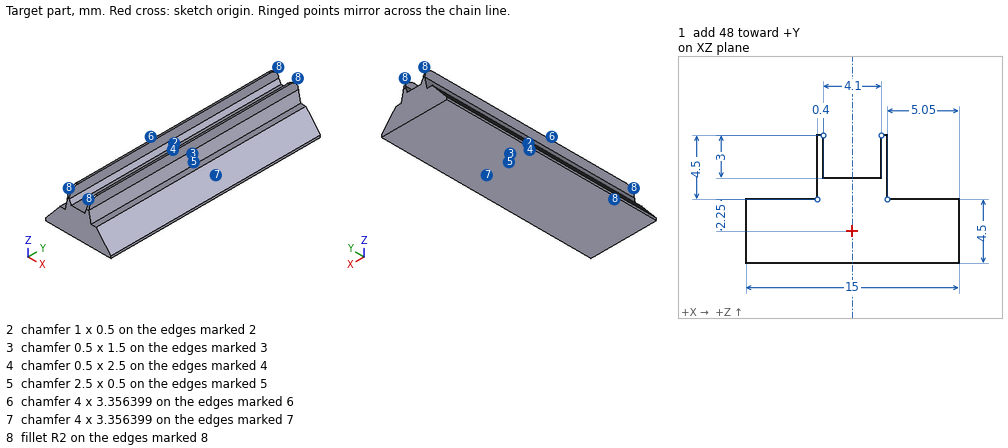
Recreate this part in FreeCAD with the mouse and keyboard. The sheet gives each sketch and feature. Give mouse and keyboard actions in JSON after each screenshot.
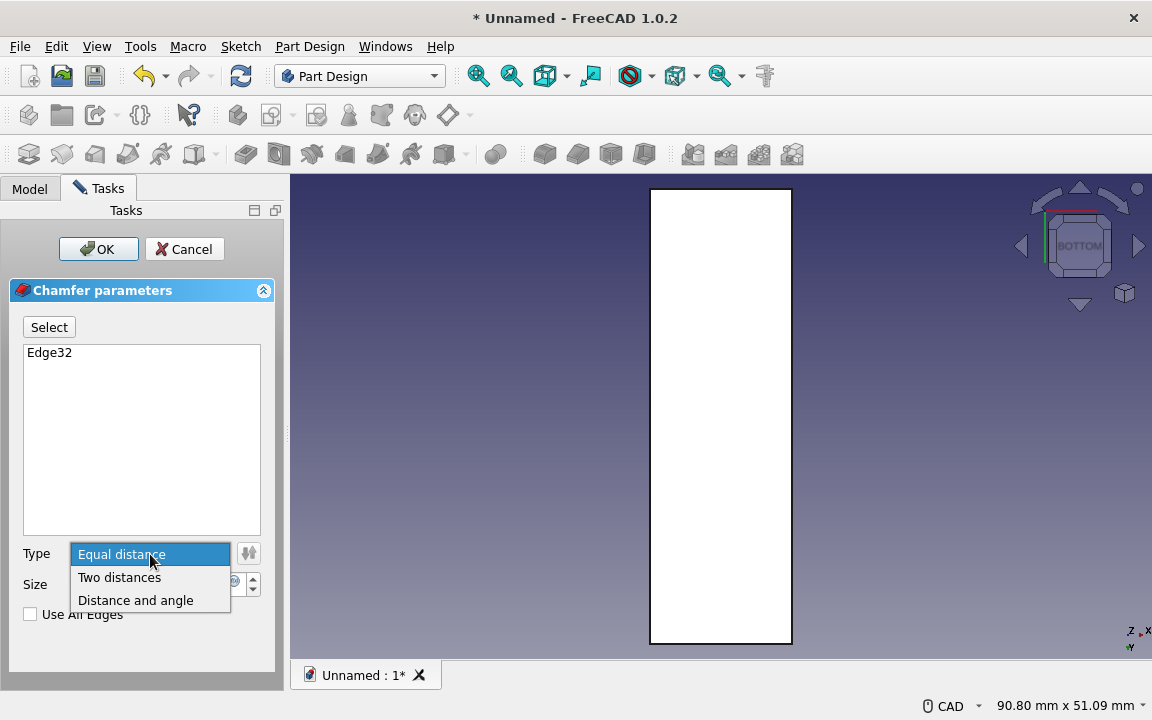
{"action": "left_click", "coordinate": [148, 578]}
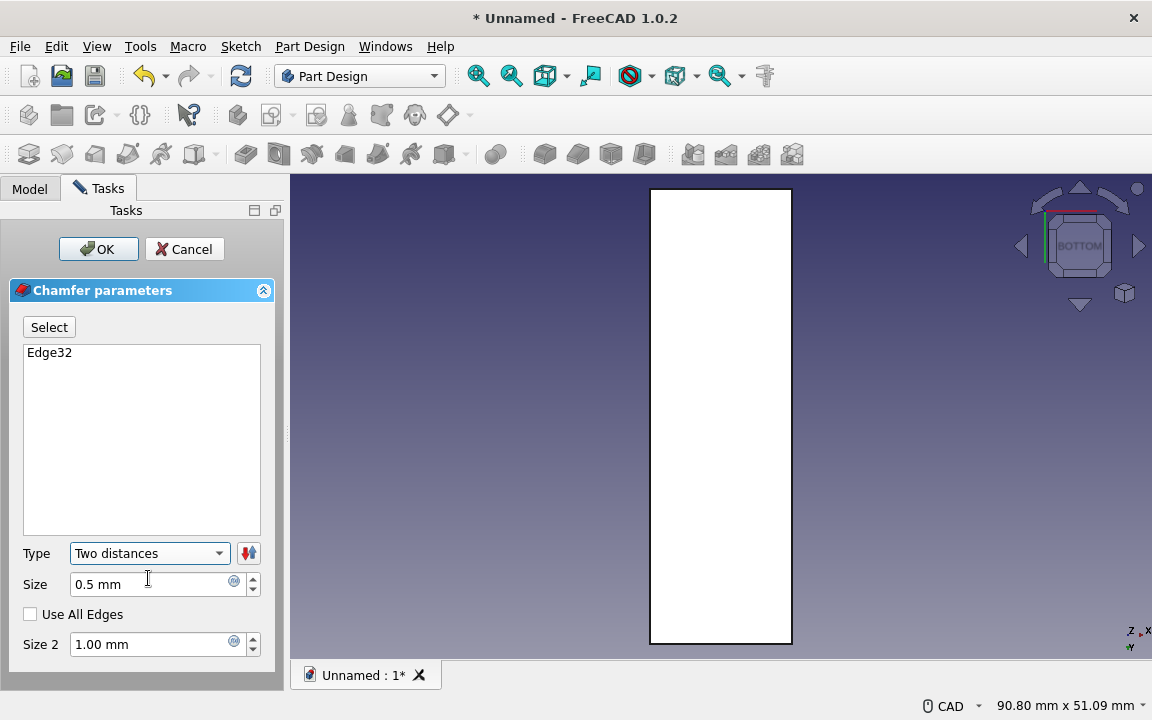
{"action": "triple_click", "coordinate": [158, 644]}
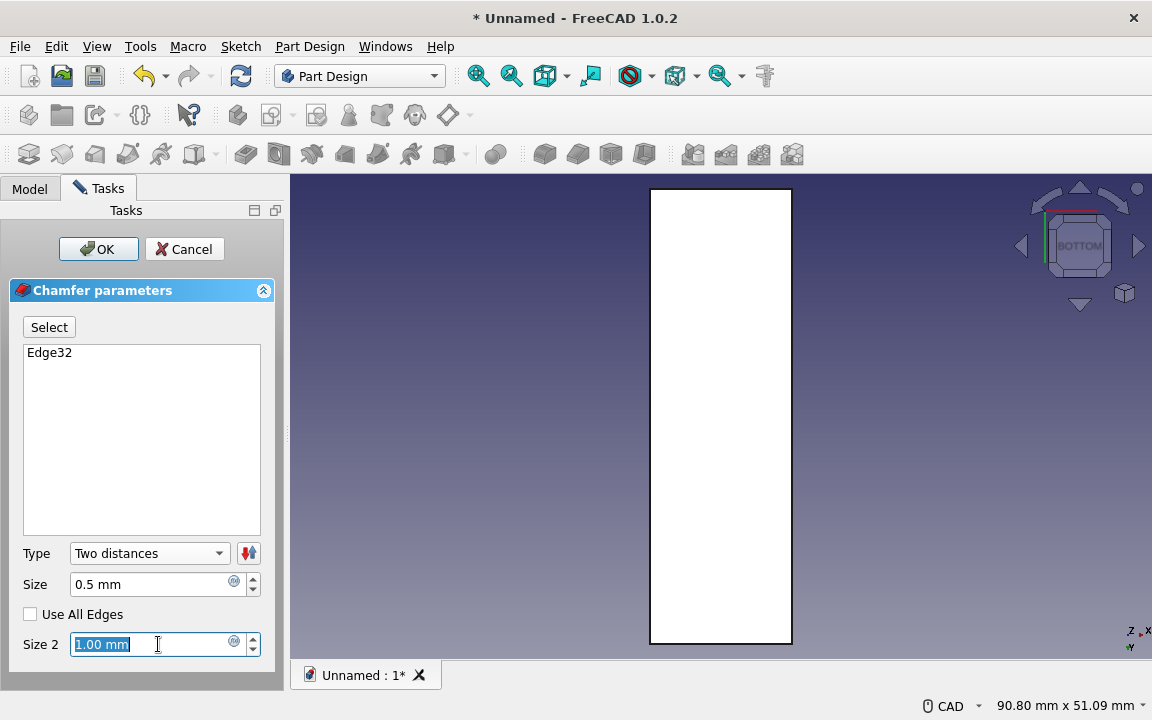
{"action": "type", "text": "2.5"}
{"action": "key", "text": "Tab"}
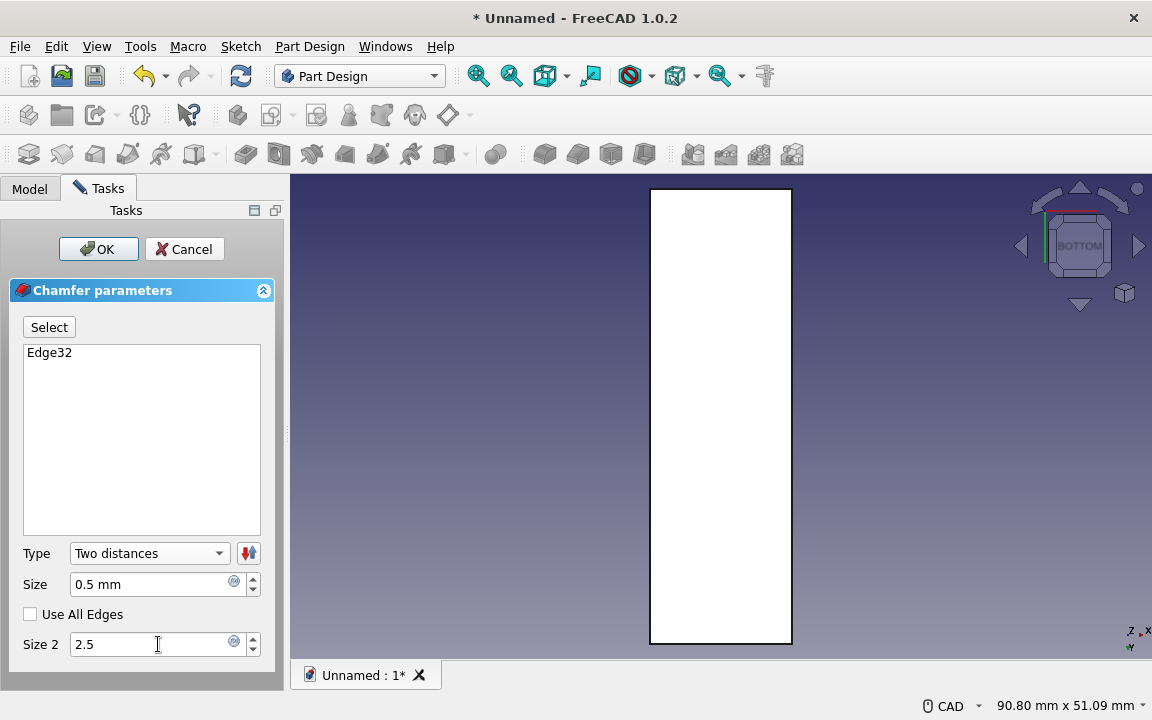
{"action": "left_click", "coordinate": [249, 554]}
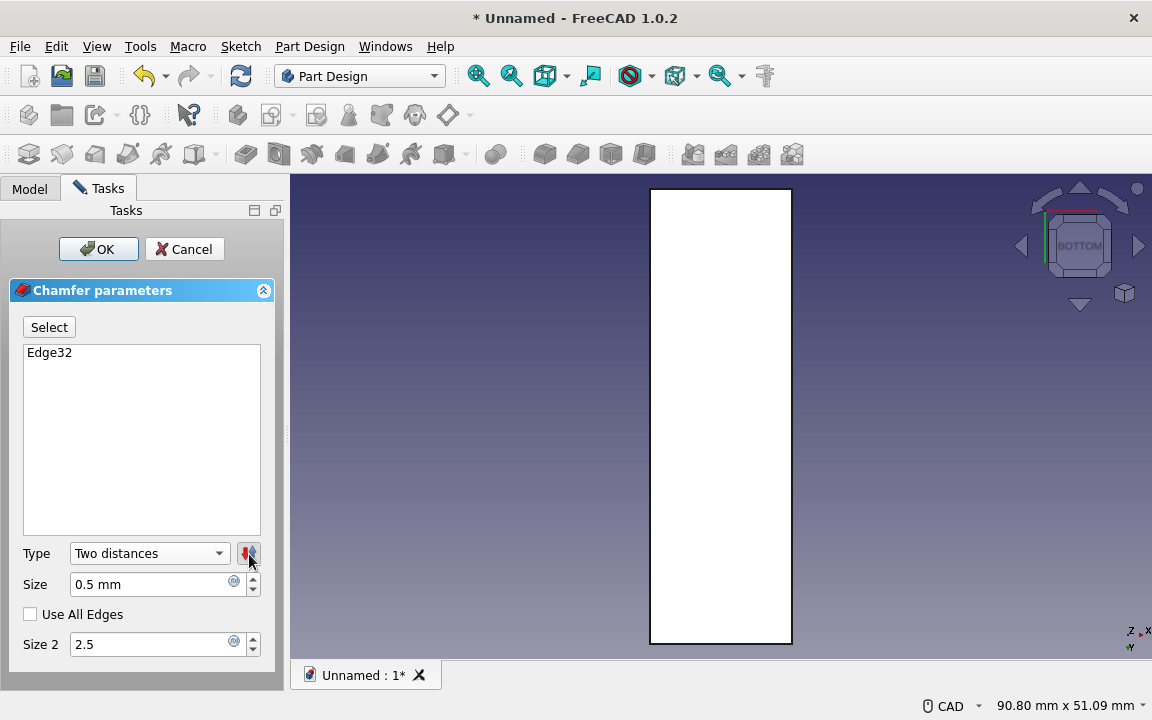
{"action": "left_click", "coordinate": [99, 249]}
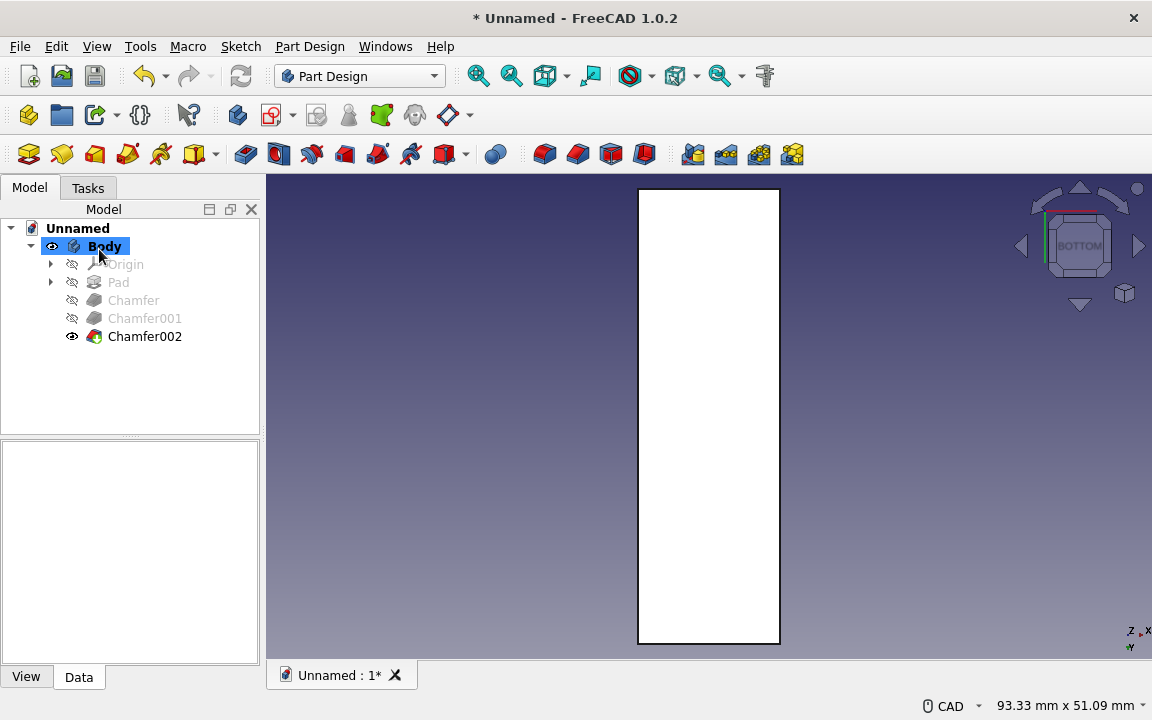
{"action": "key", "text": "0"}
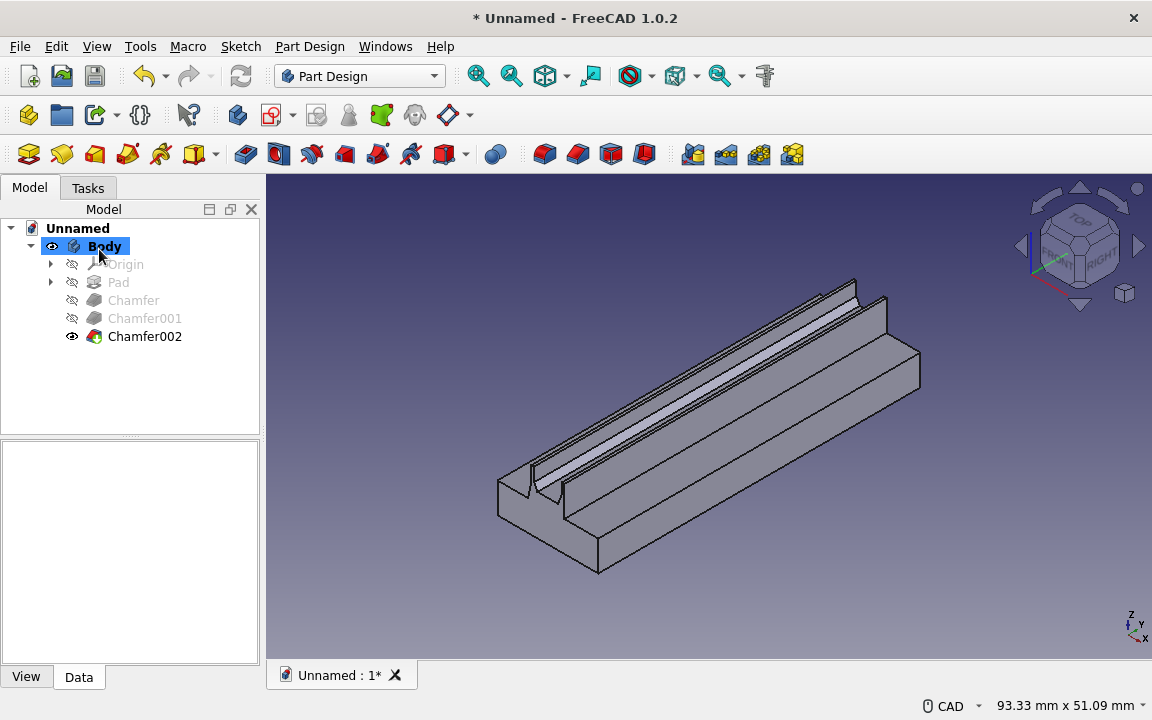
{"action": "key", "text": "2"}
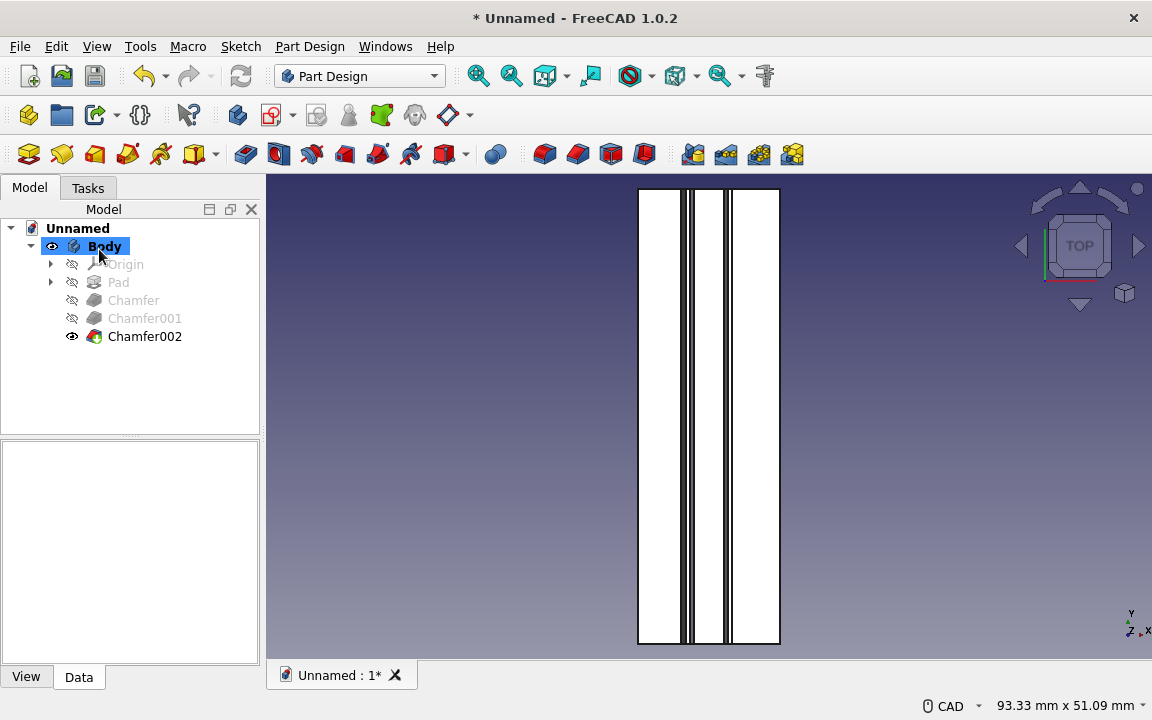
{"action": "key", "text": "1"}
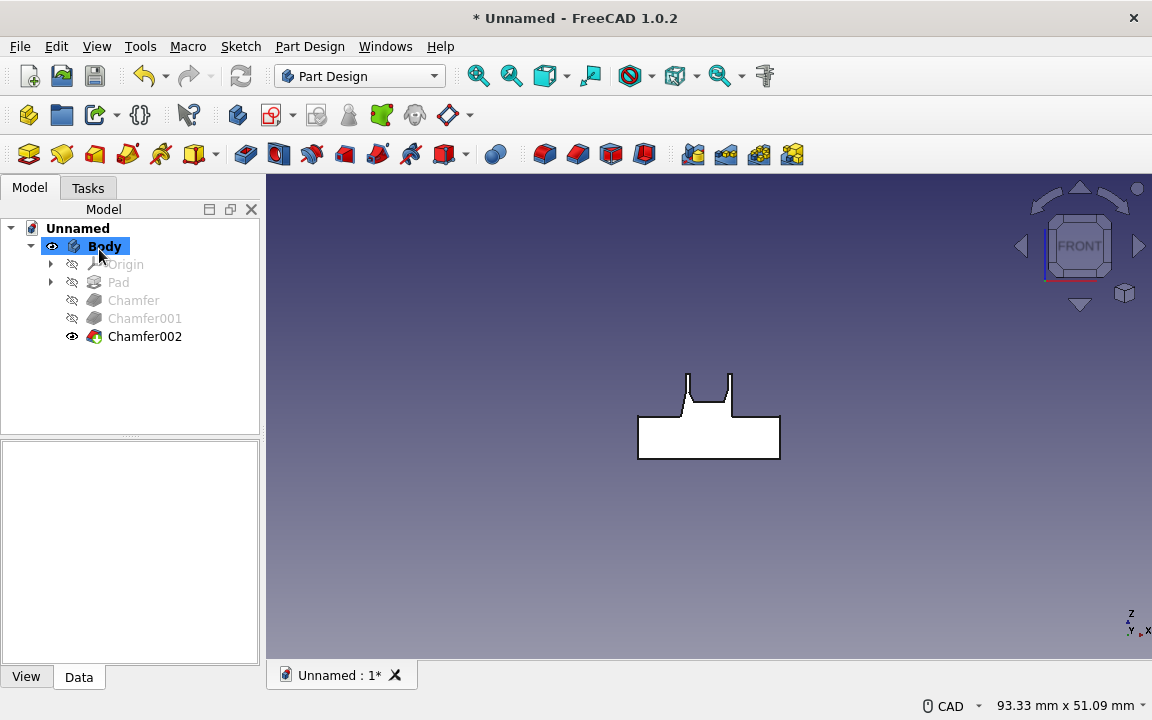
{"action": "left_click", "coordinate": [479, 76]}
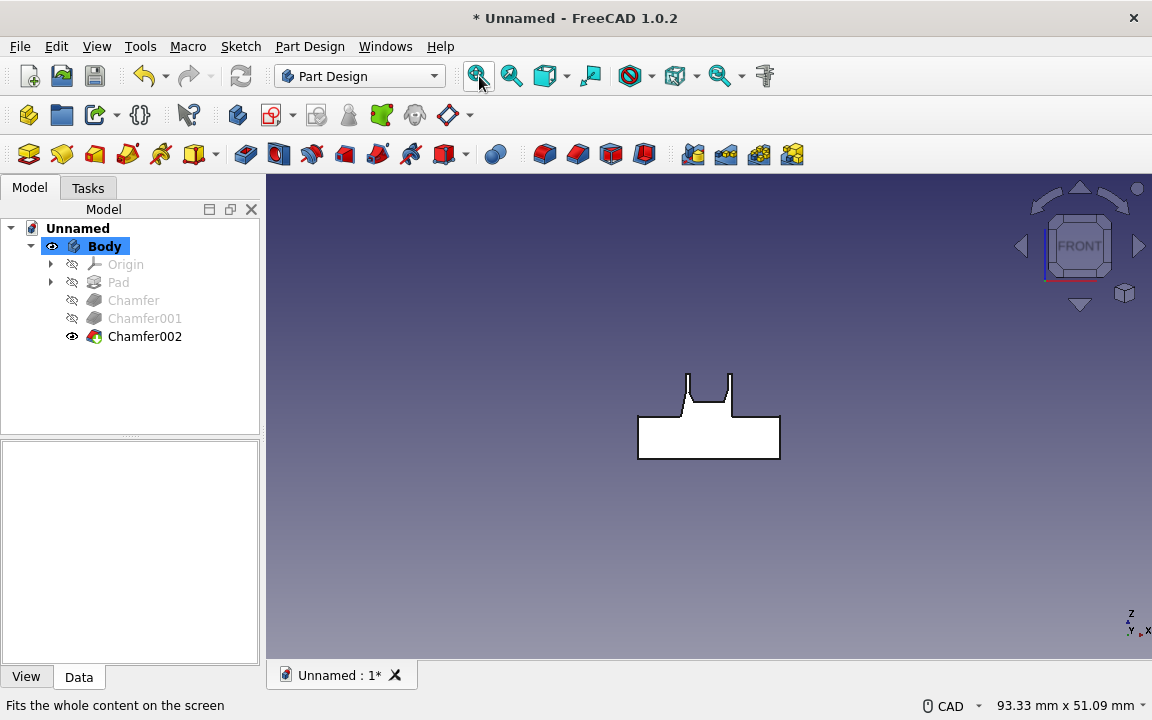
{"action": "key", "text": "3"}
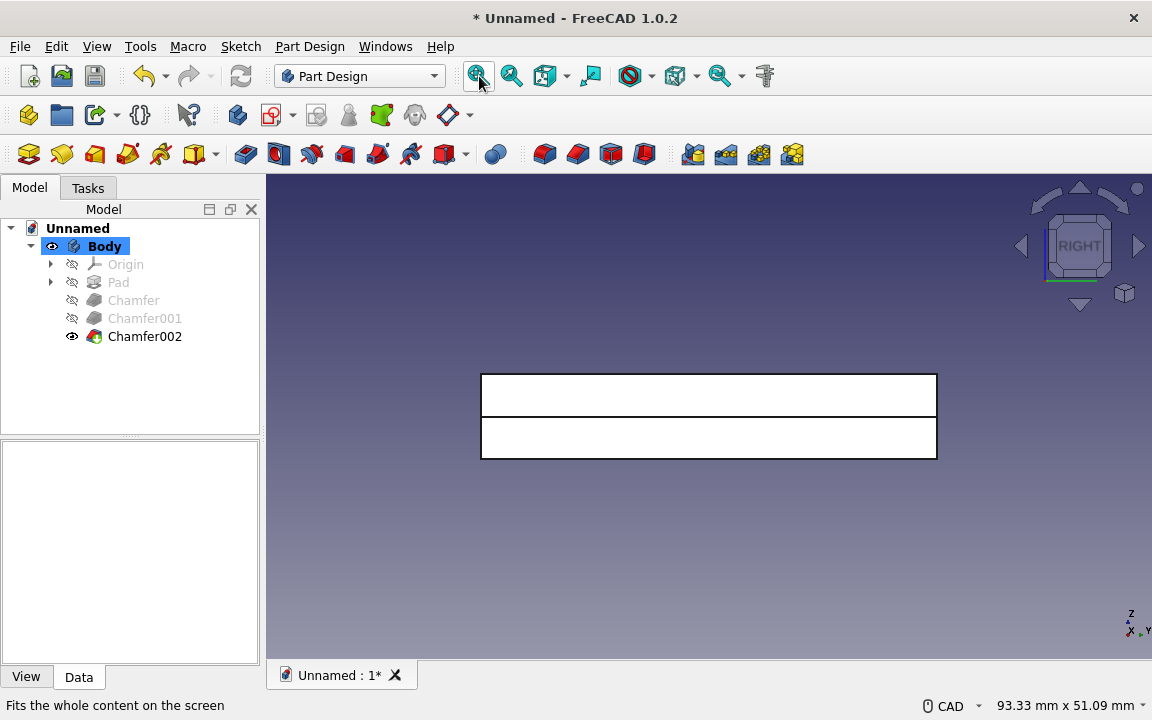
{"action": "key", "text": "5"}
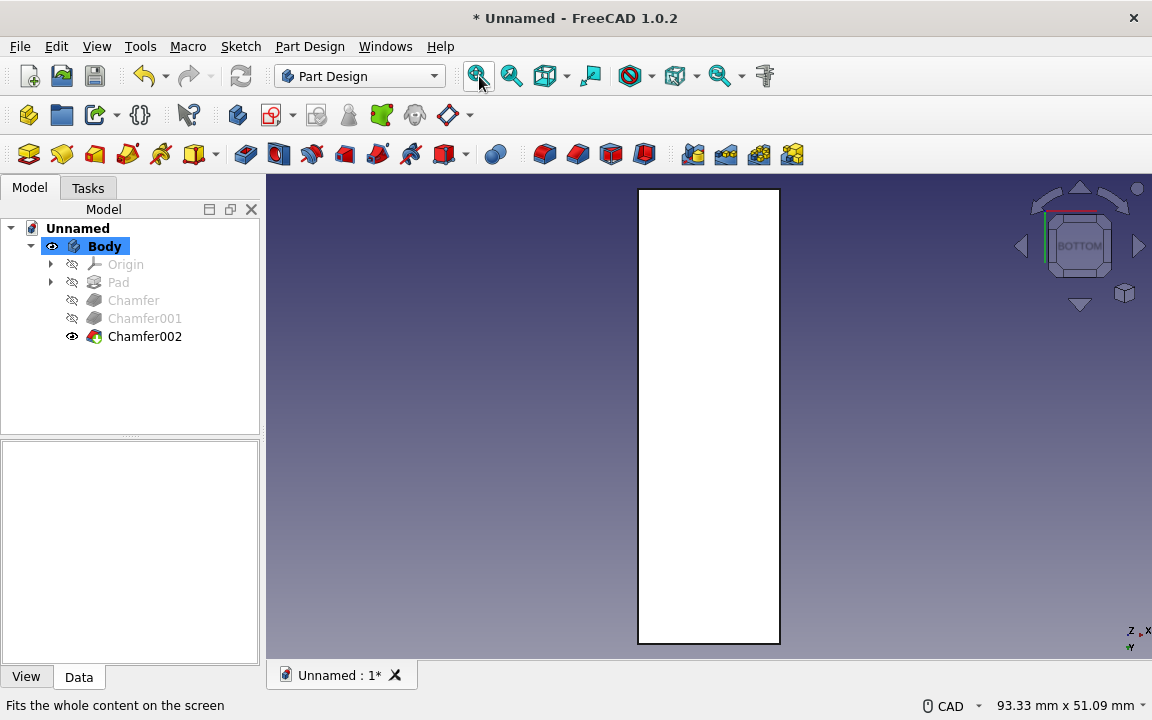
{"action": "key", "text": "4"}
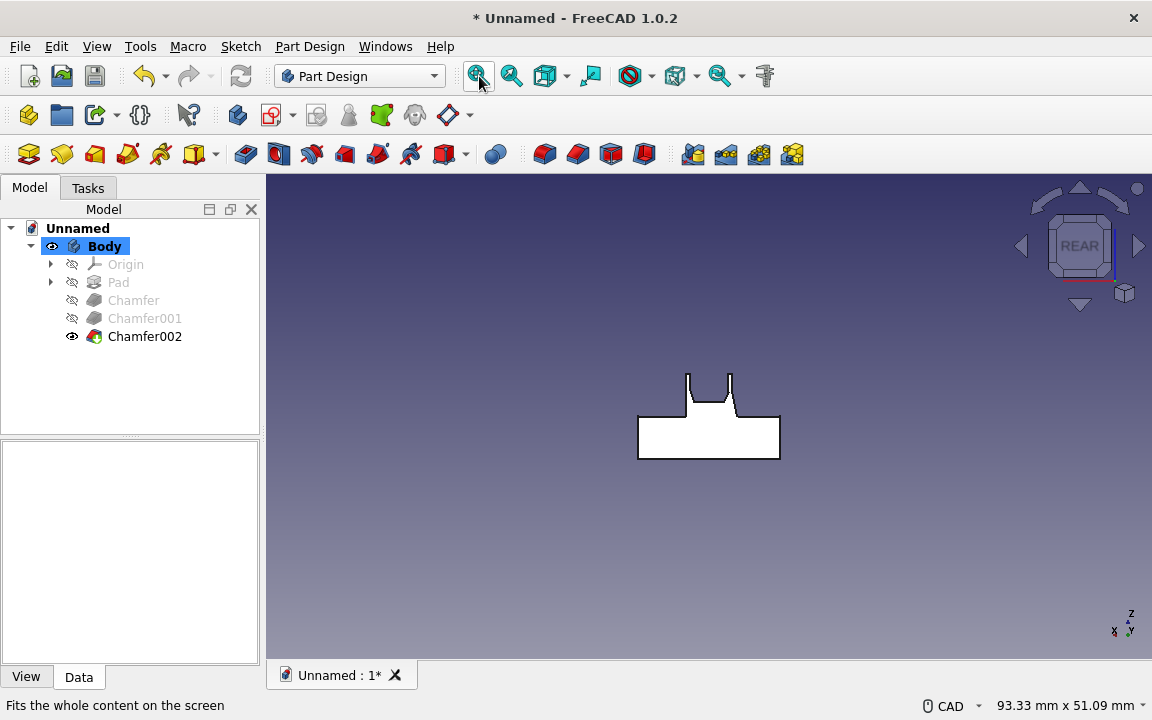
{"action": "left_click", "coordinate": [479, 76]}